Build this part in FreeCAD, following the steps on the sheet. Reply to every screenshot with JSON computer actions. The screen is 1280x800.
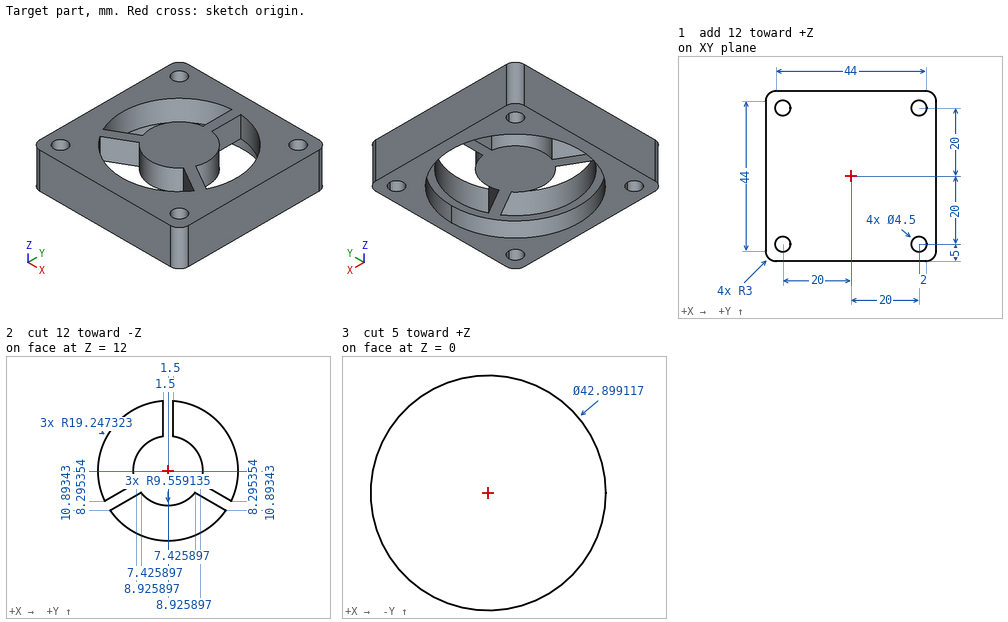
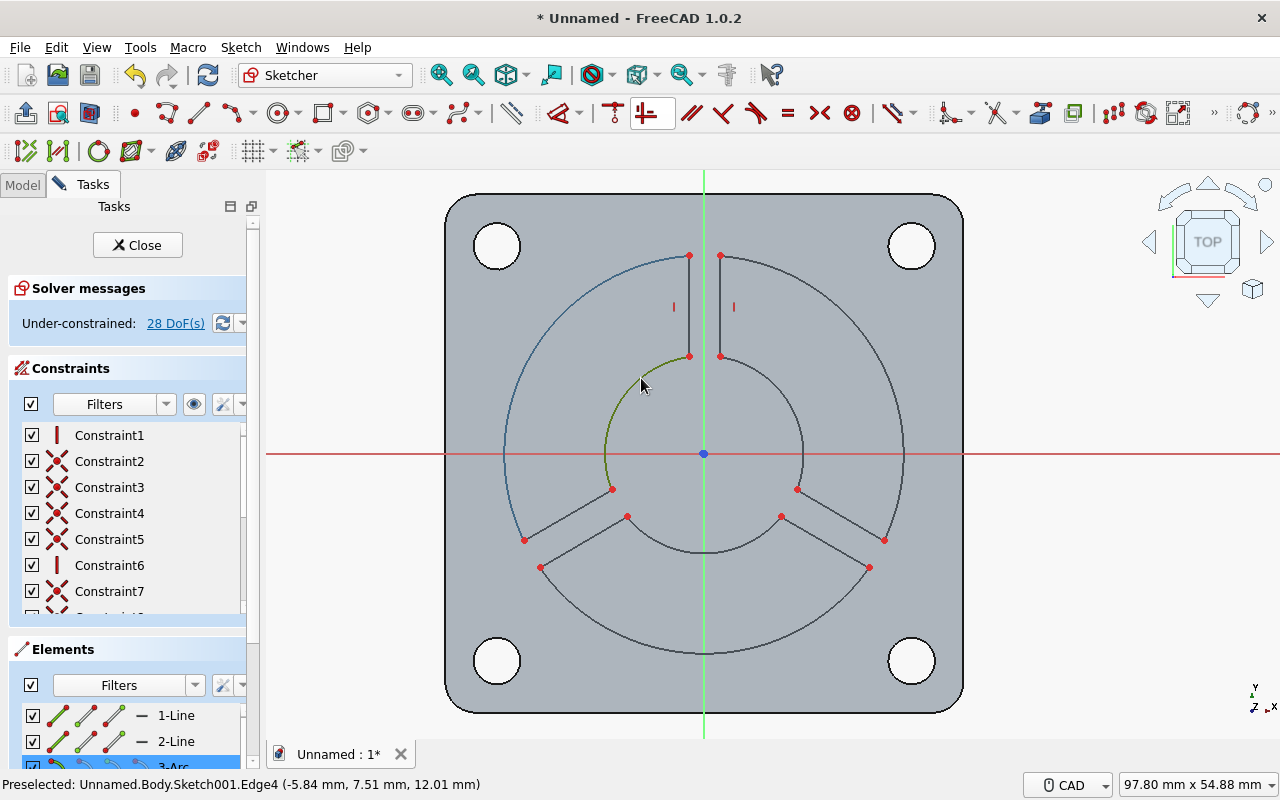
{"action": "left_click", "coordinate": [614, 114]}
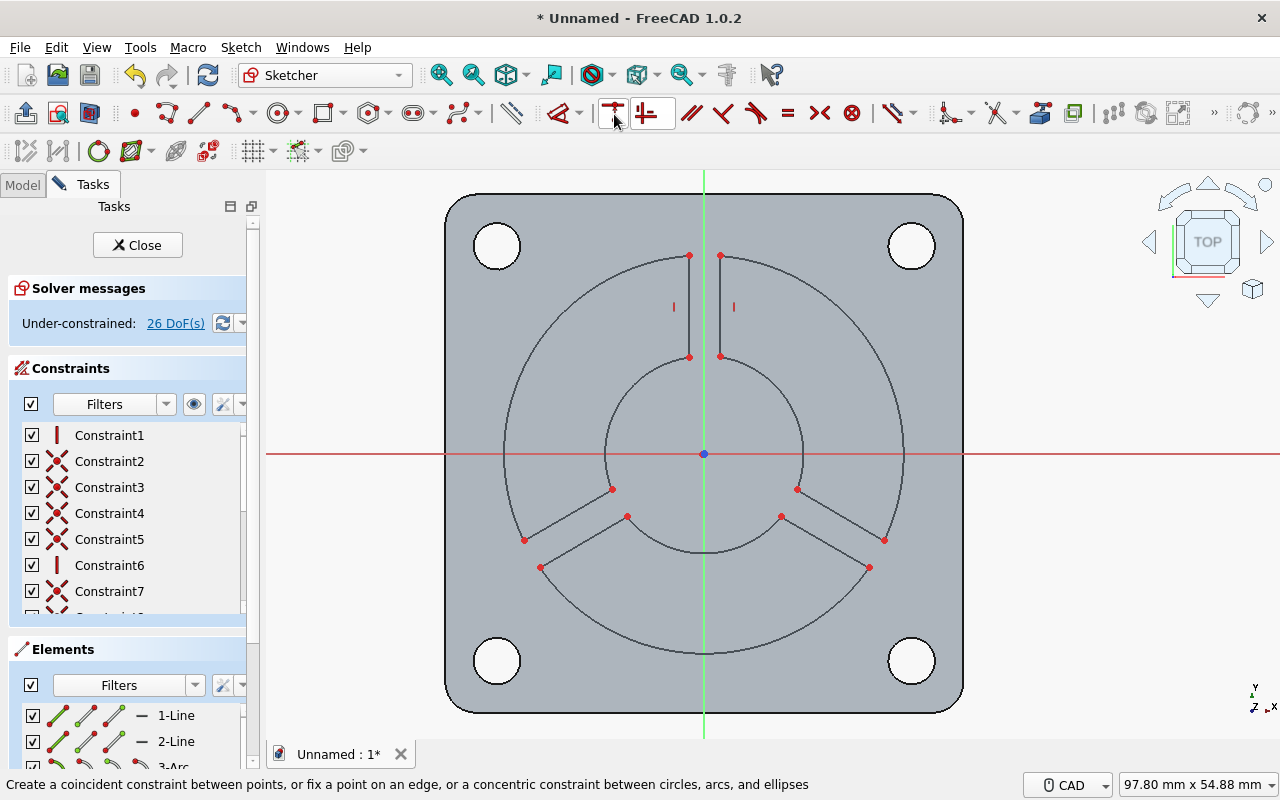
{"action": "left_click", "coordinate": [582, 297]}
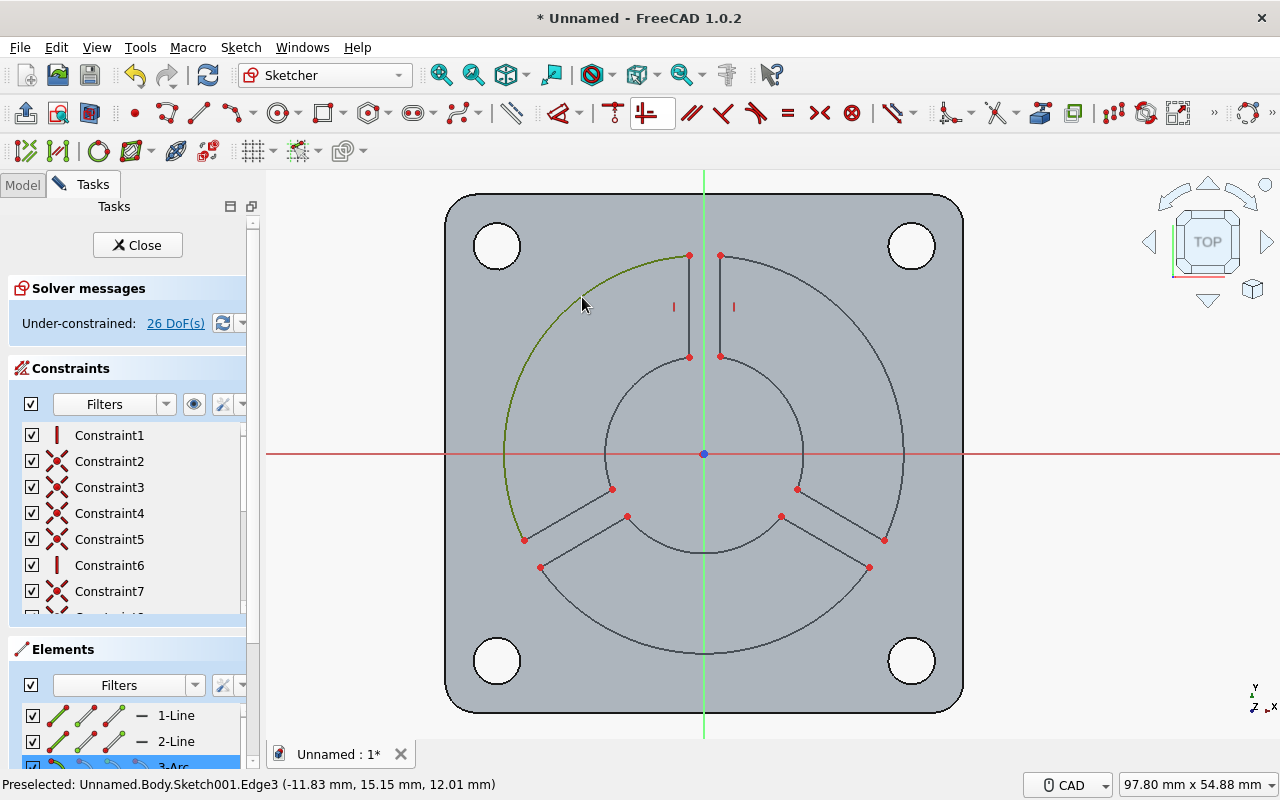
{"action": "left_click", "coordinate": [802, 438]}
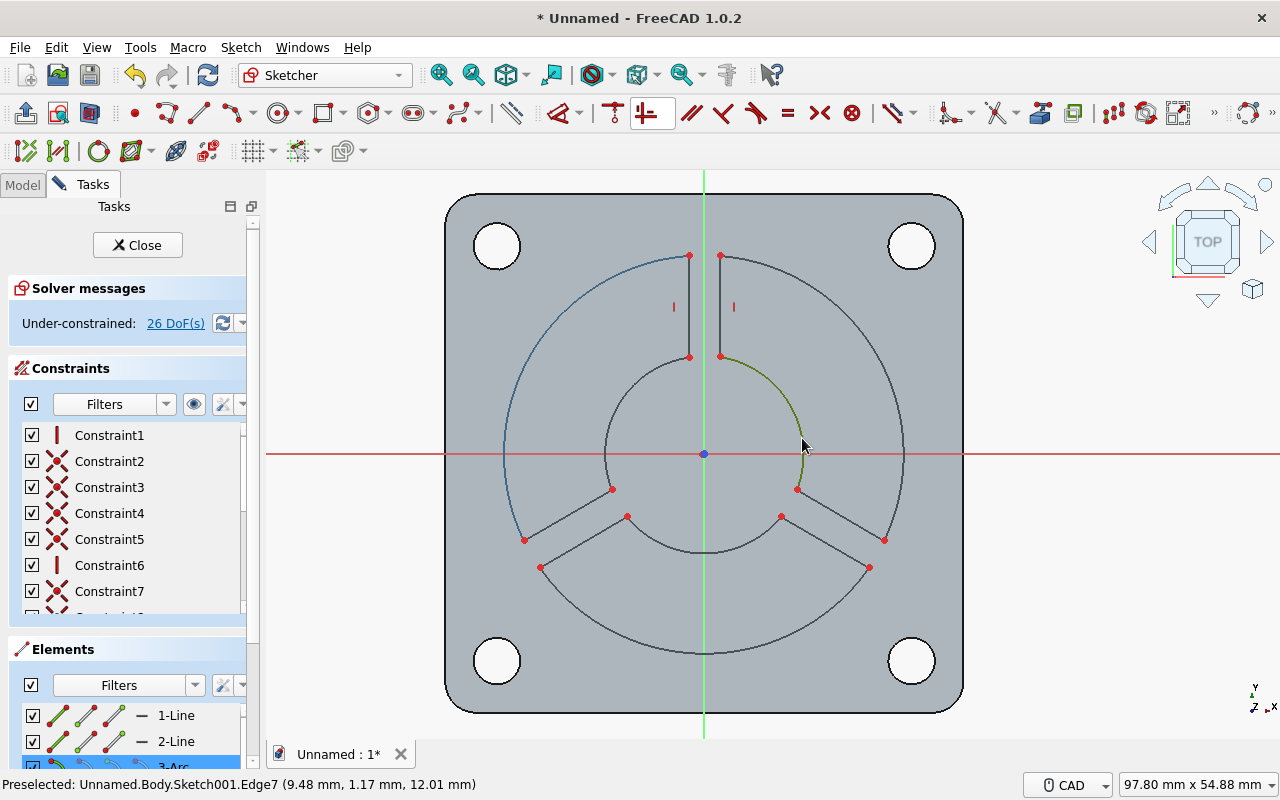
{"action": "left_click", "coordinate": [614, 114]}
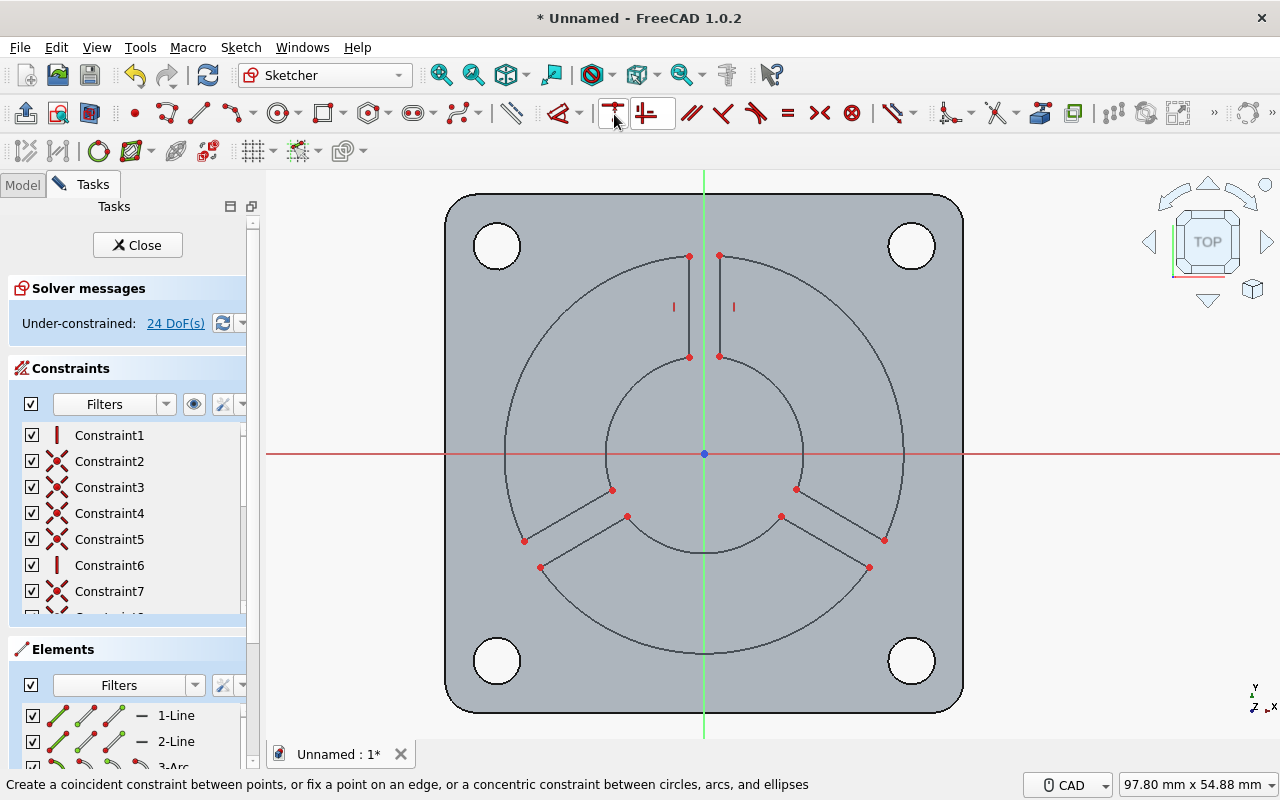
{"action": "left_click", "coordinate": [582, 297]}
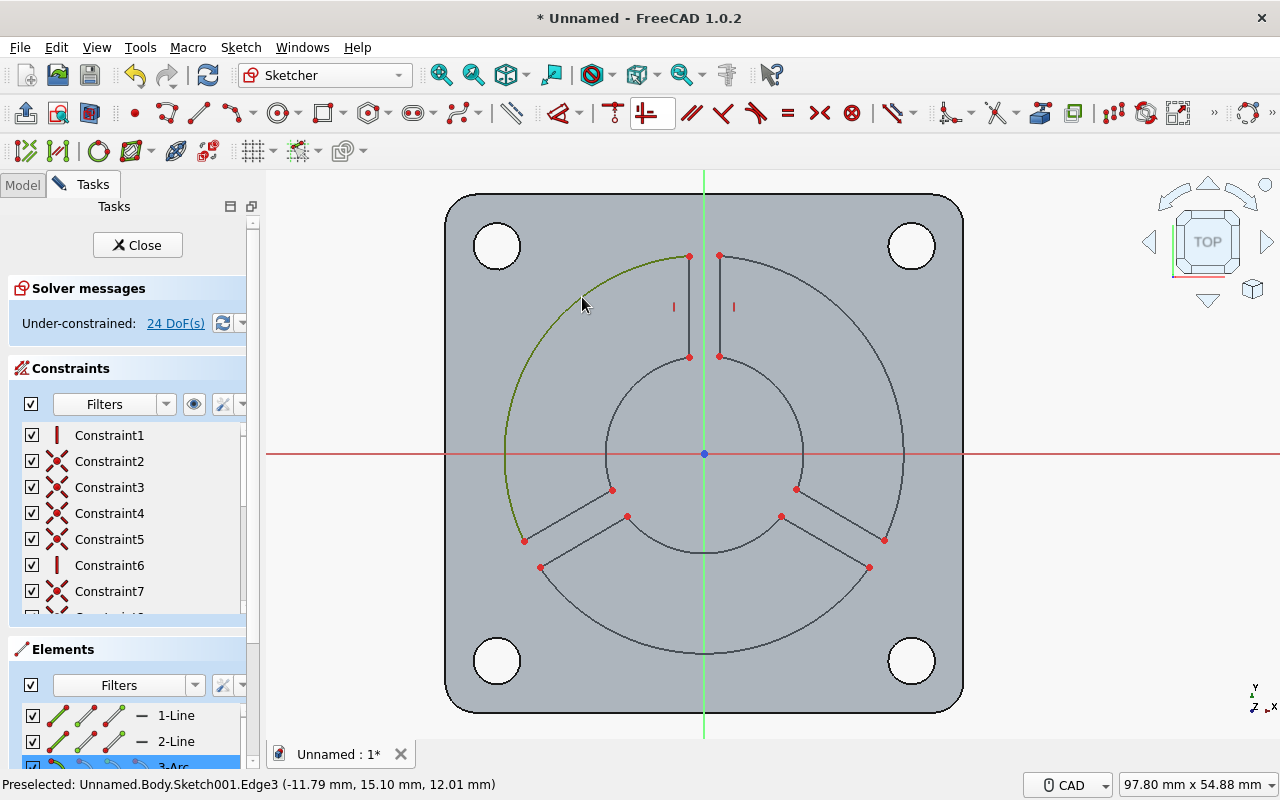
{"action": "left_click", "coordinate": [902, 428]}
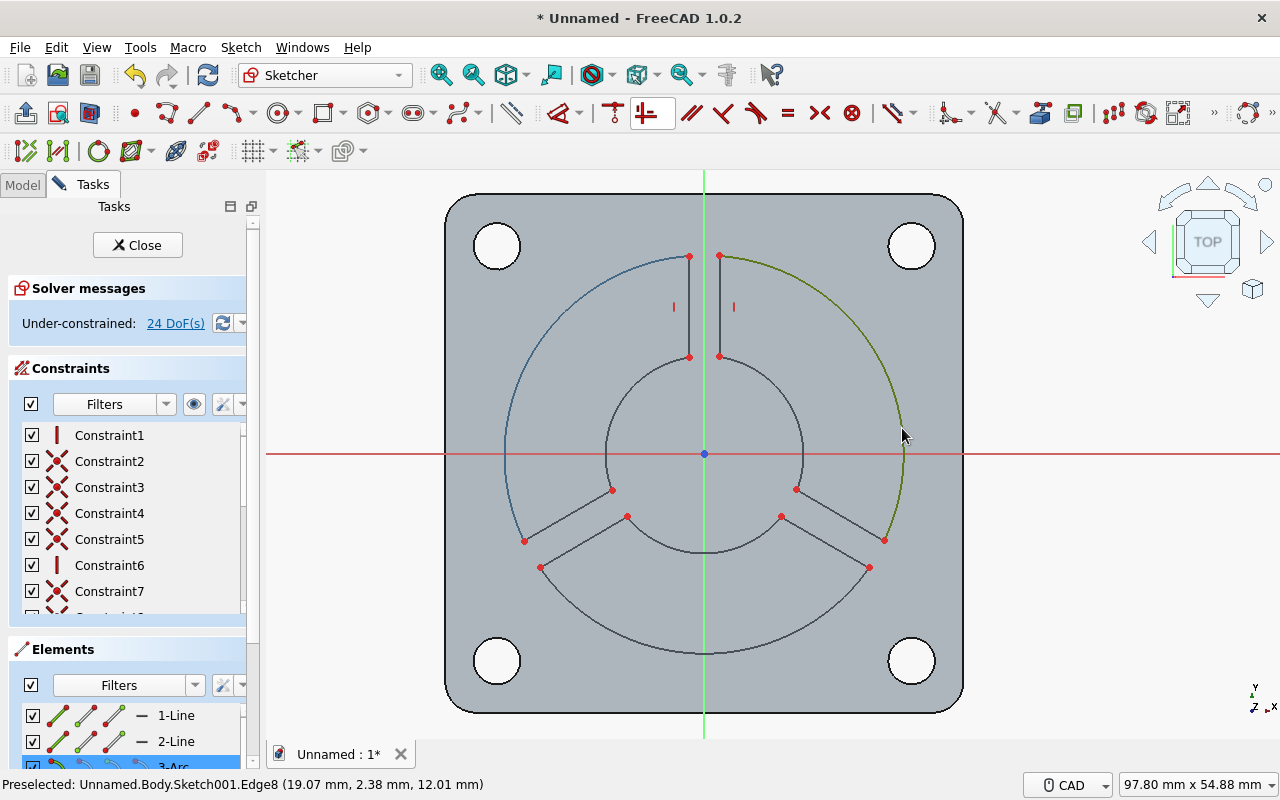
{"action": "left_click", "coordinate": [614, 114]}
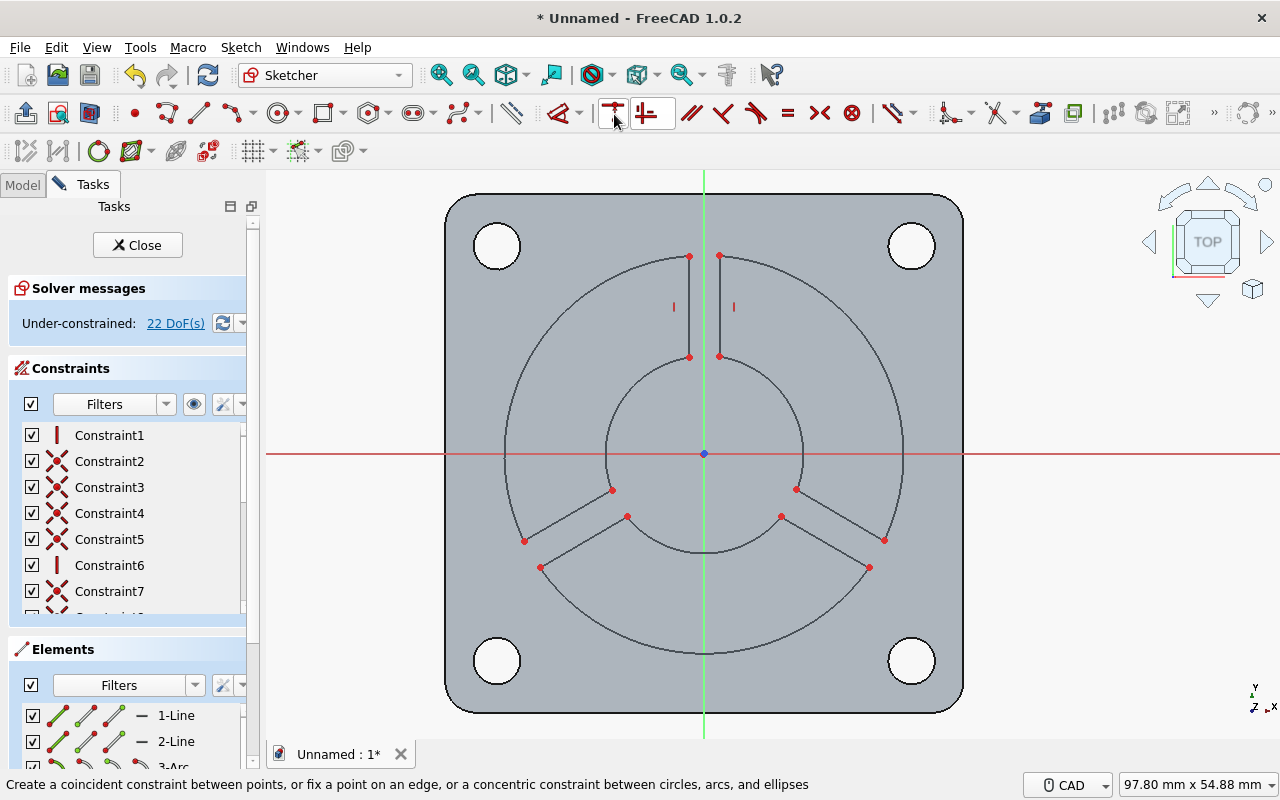
{"action": "left_click", "coordinate": [582, 297]}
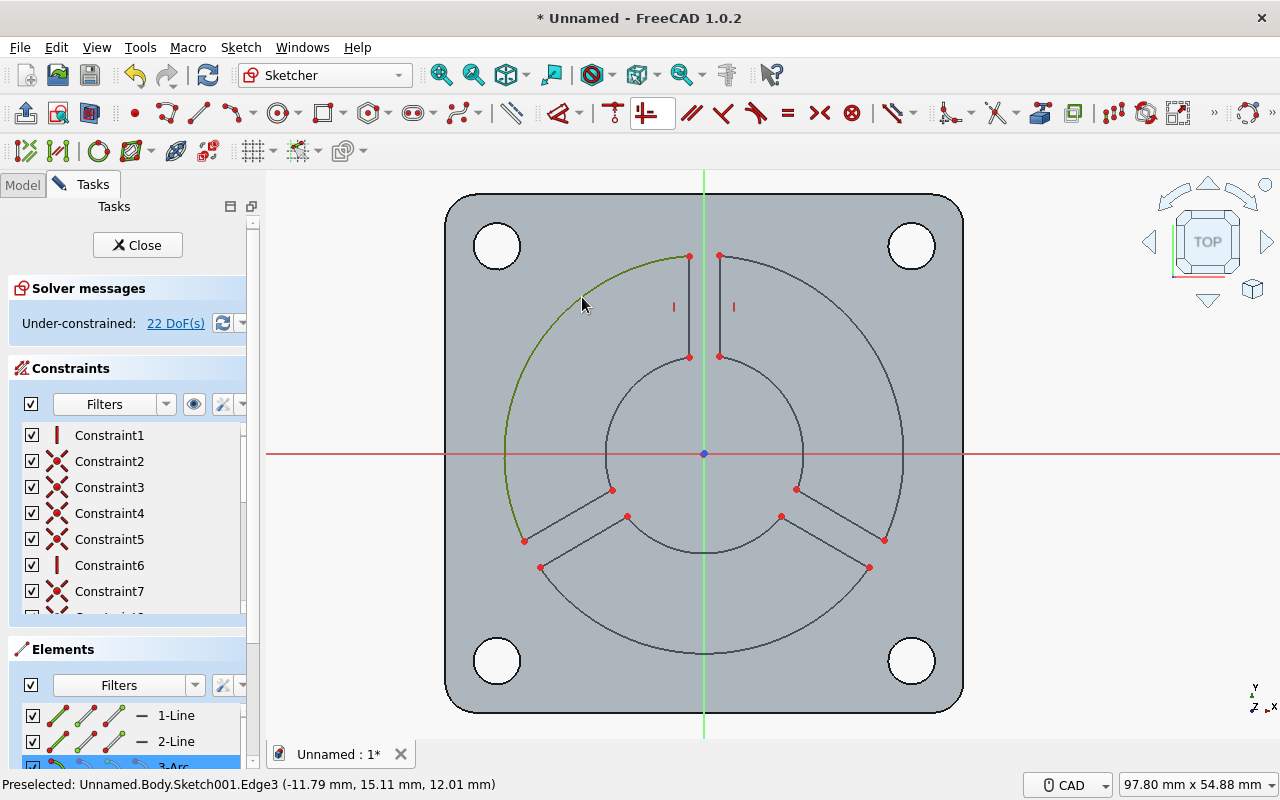
{"action": "left_click", "coordinate": [670, 547]}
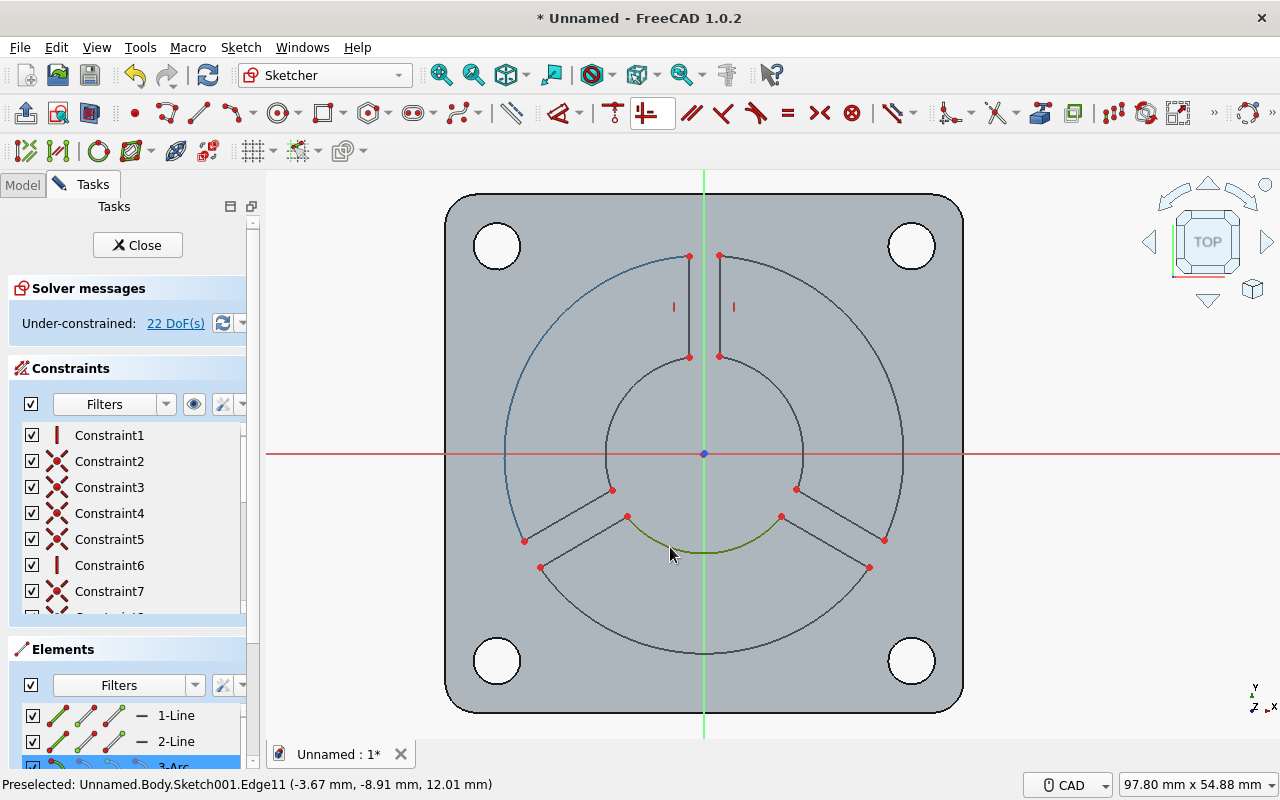
{"action": "left_click", "coordinate": [614, 114]}